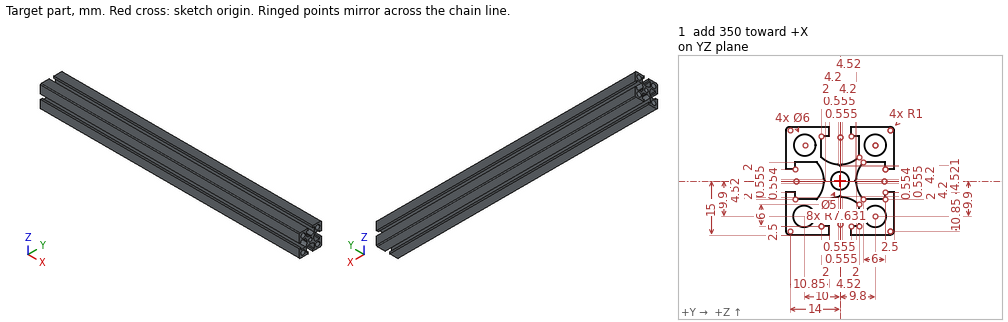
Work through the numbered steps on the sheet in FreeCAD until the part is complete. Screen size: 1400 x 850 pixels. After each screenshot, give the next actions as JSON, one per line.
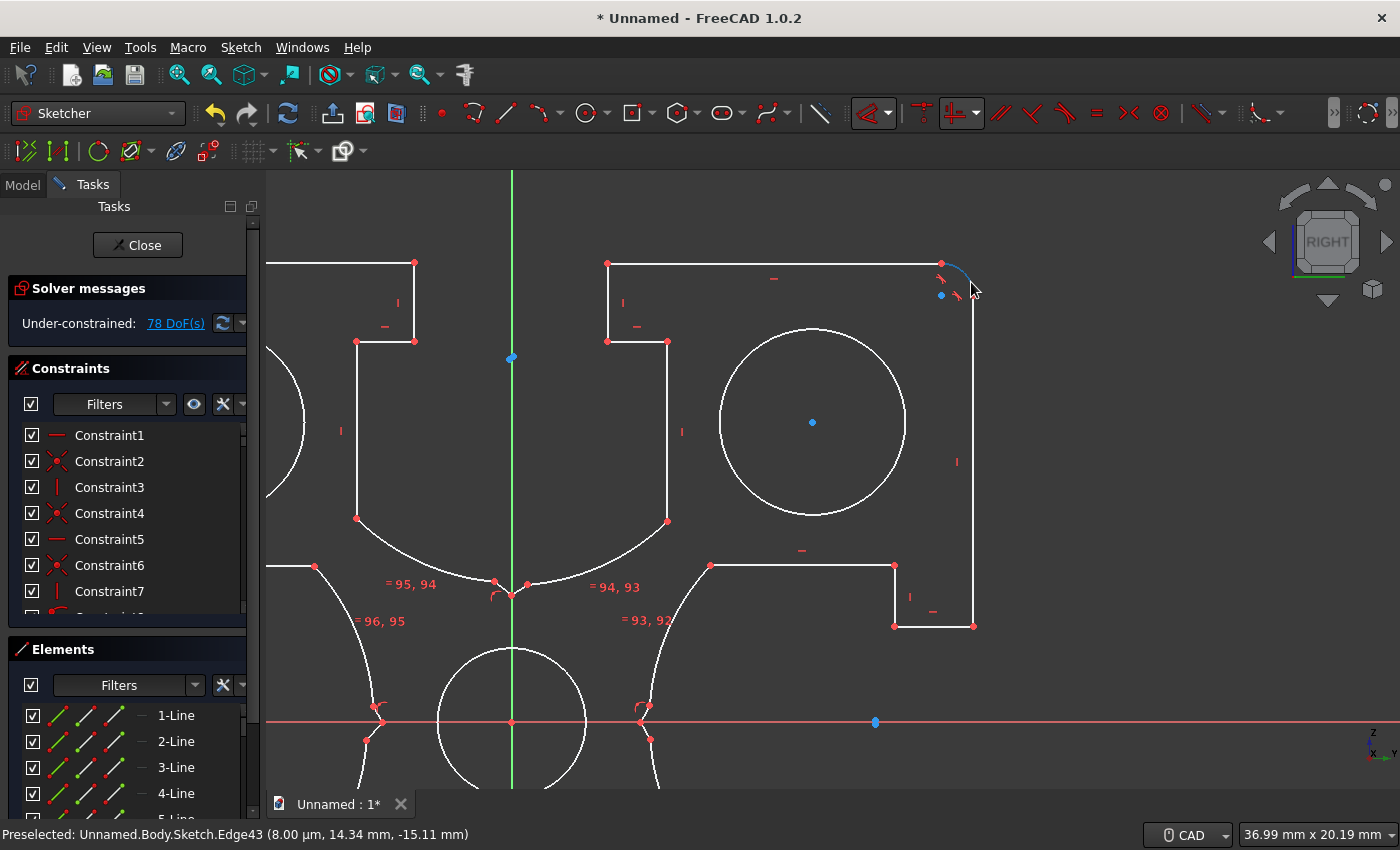
{"action": "left_click", "coordinate": [970, 281]}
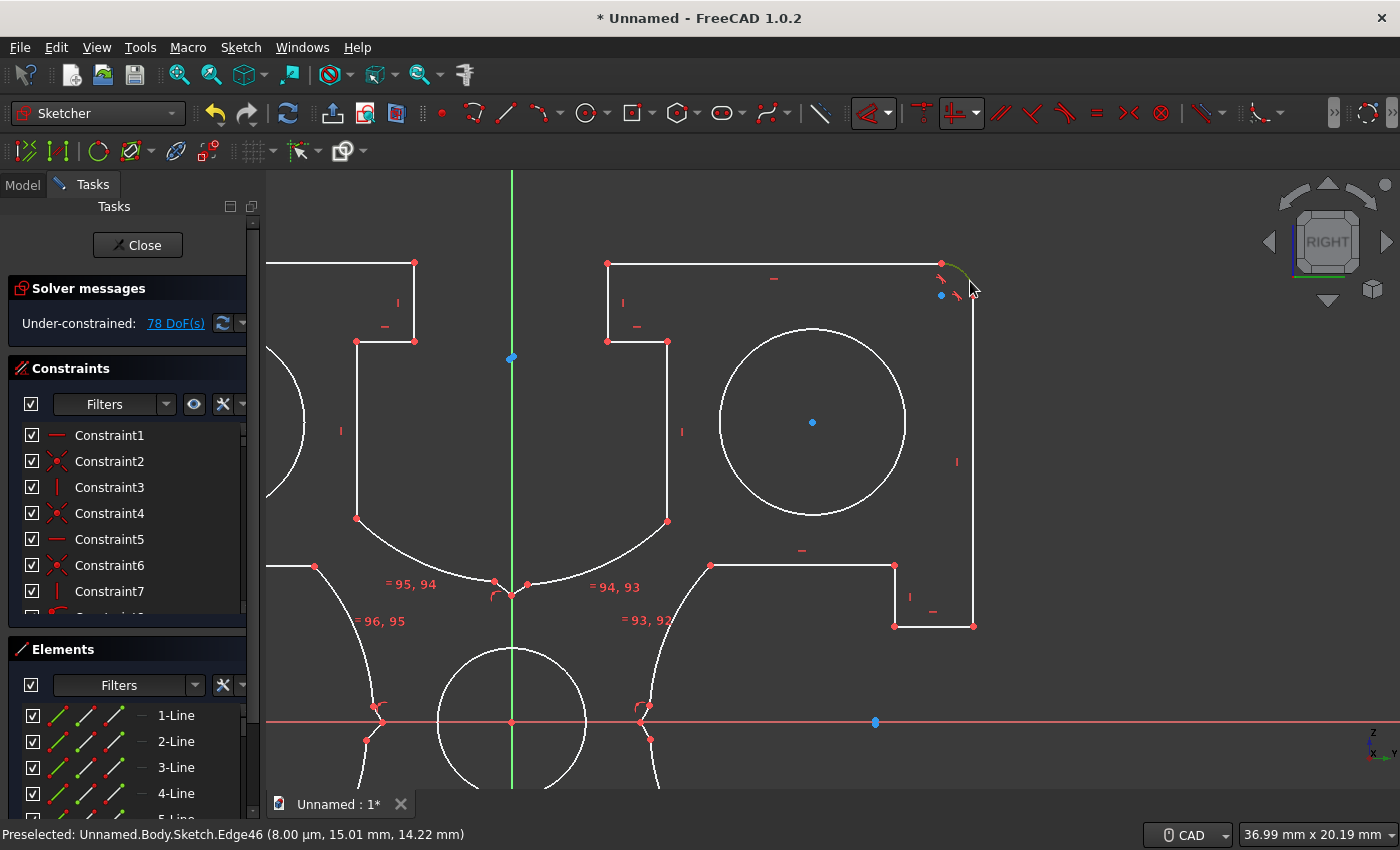
{"action": "scroll", "coordinate": [971, 281], "scroll_direction": "down", "scroll_amount": 4}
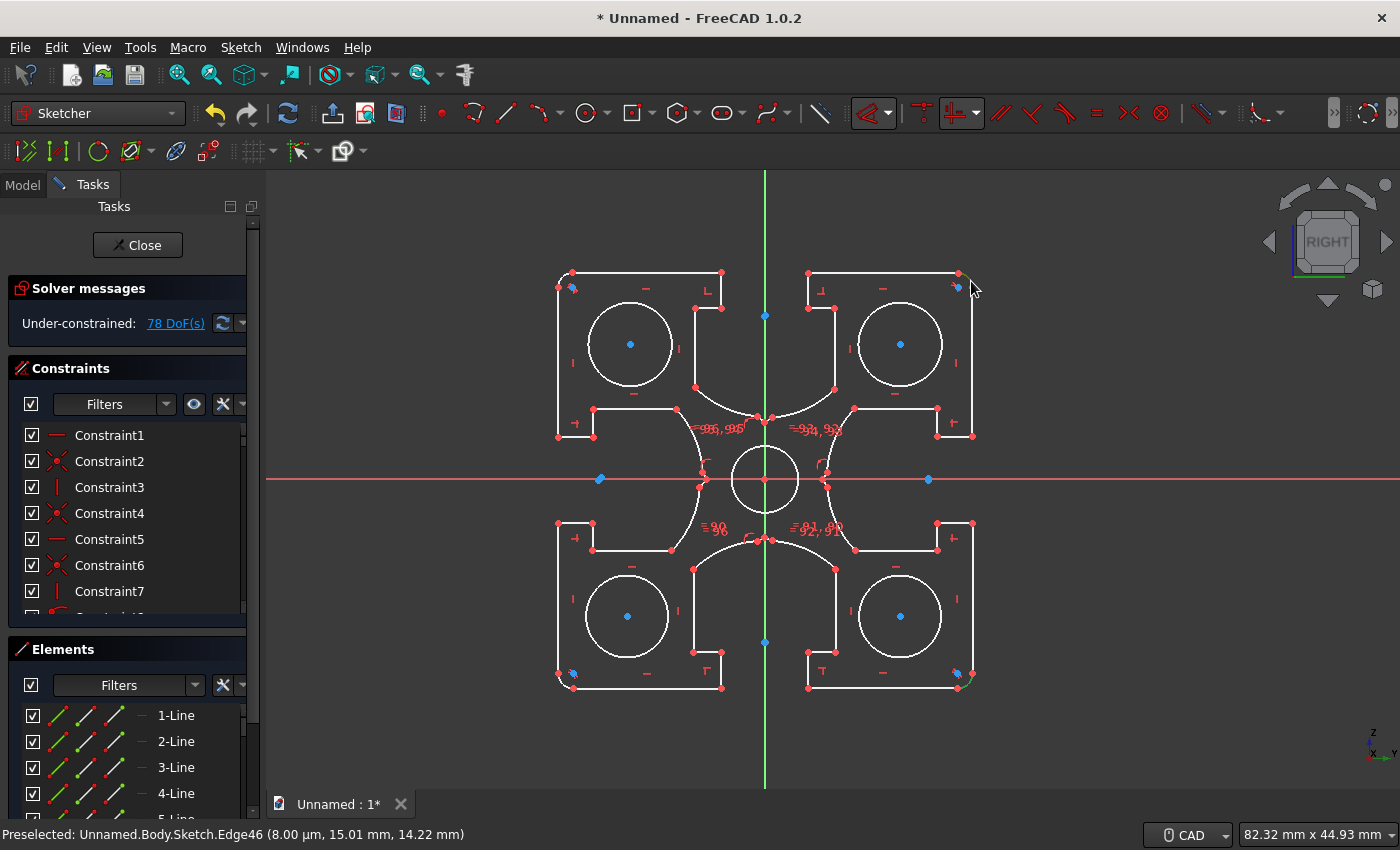
{"action": "scroll", "coordinate": [566, 274], "scroll_direction": "up", "scroll_amount": 4}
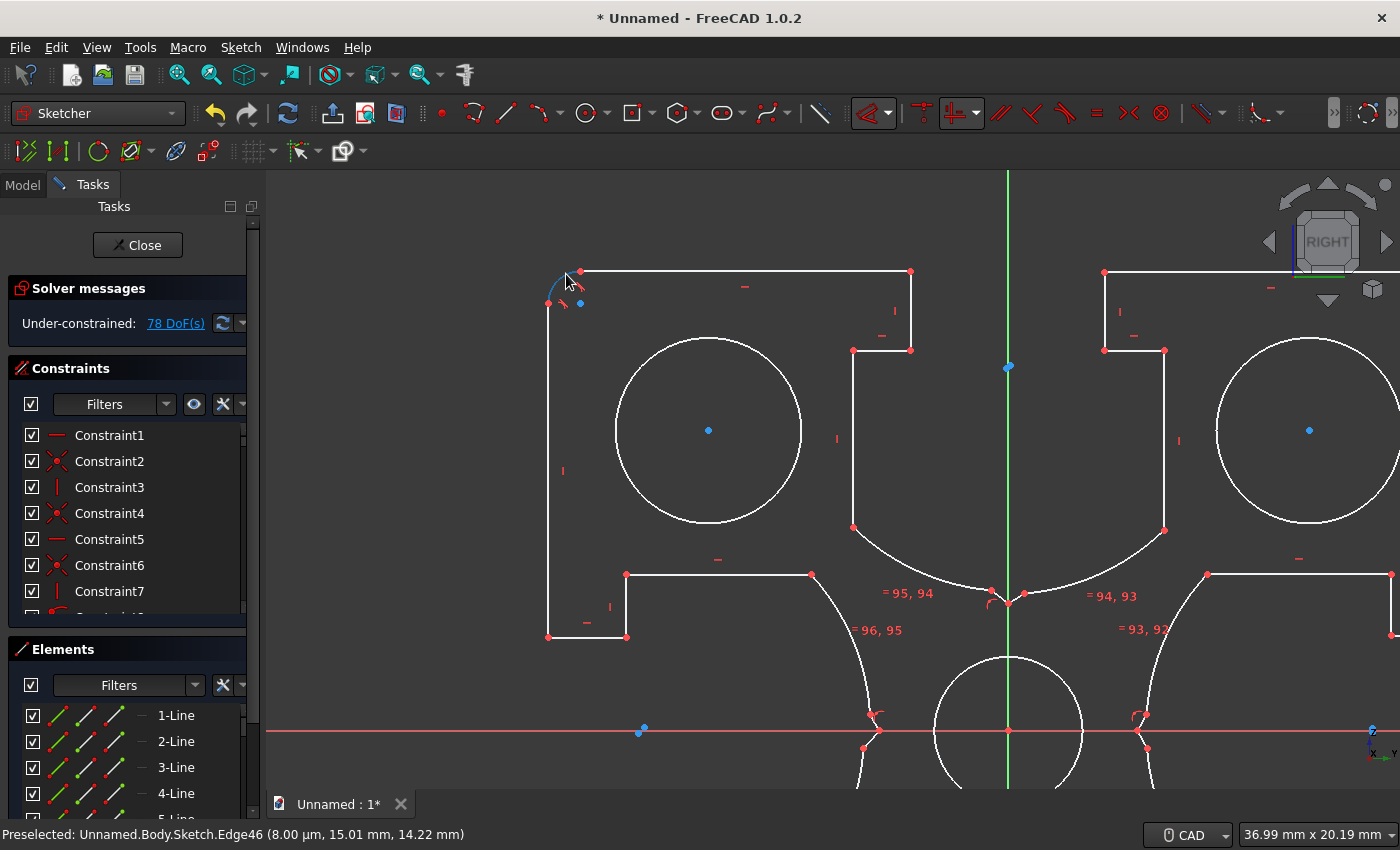
{"action": "left_click", "coordinate": [566, 275]}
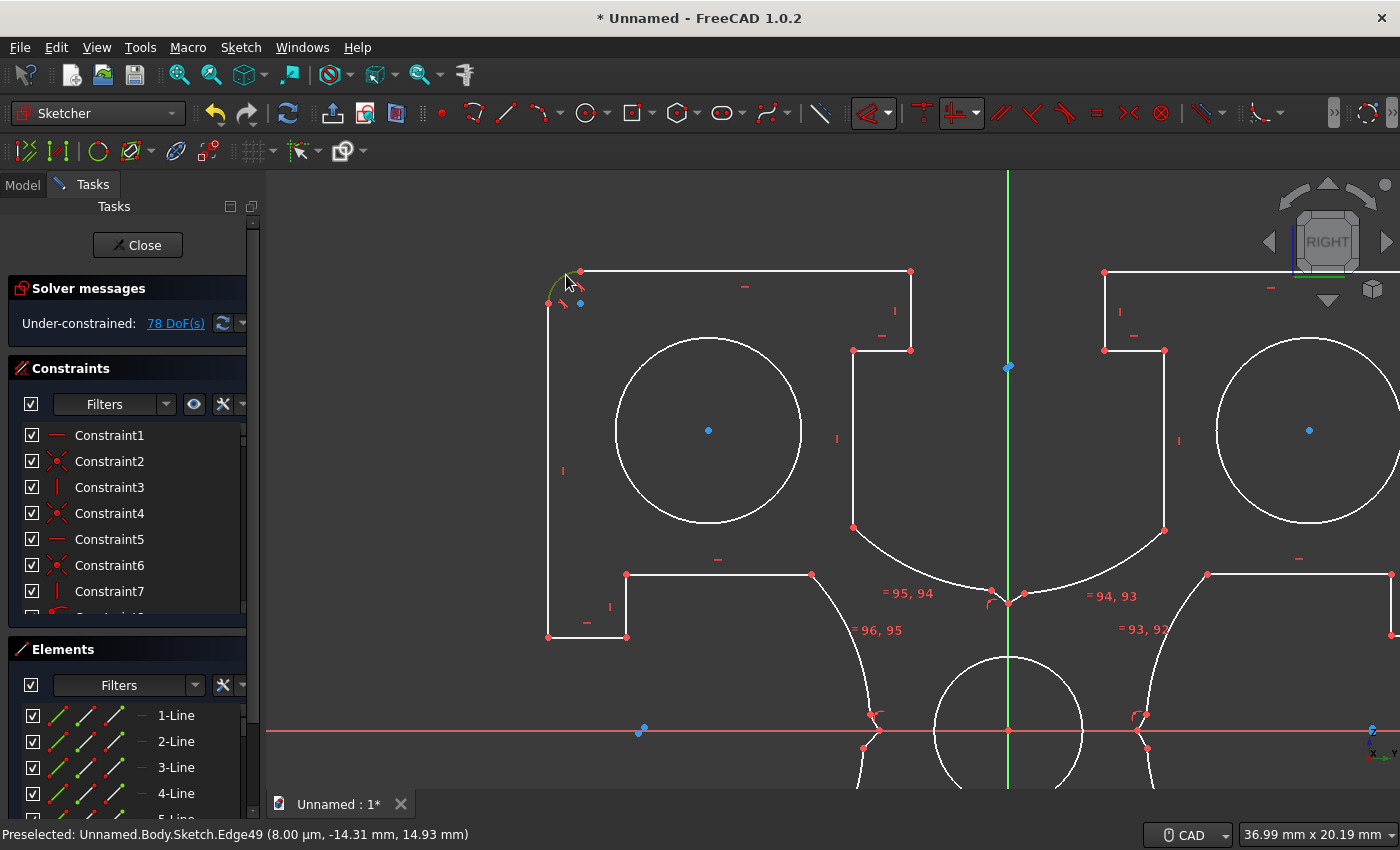
{"action": "scroll", "coordinate": [565, 274], "scroll_direction": "down", "scroll_amount": 4}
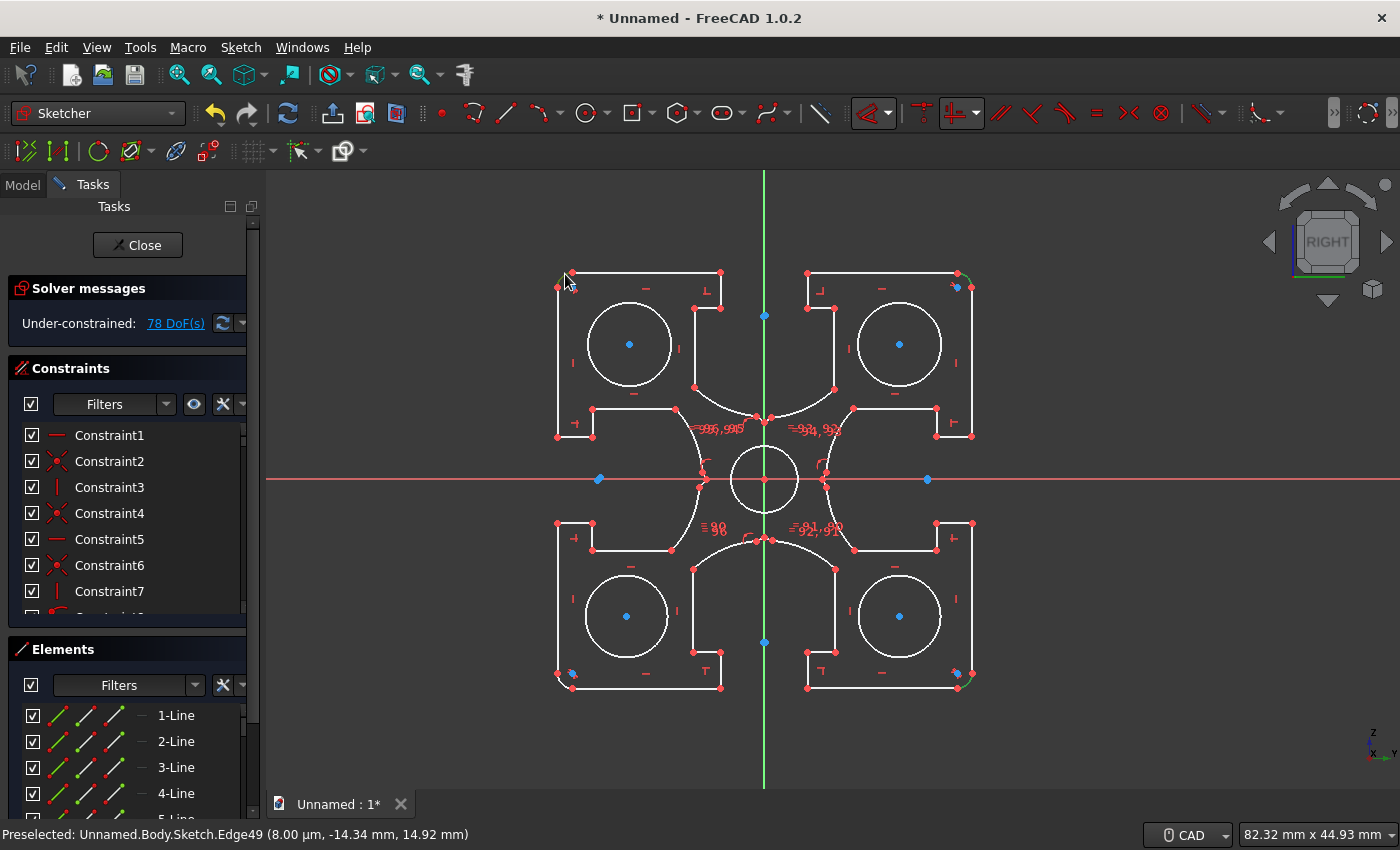
{"action": "scroll", "coordinate": [559, 680], "scroll_direction": "up", "scroll_amount": 4}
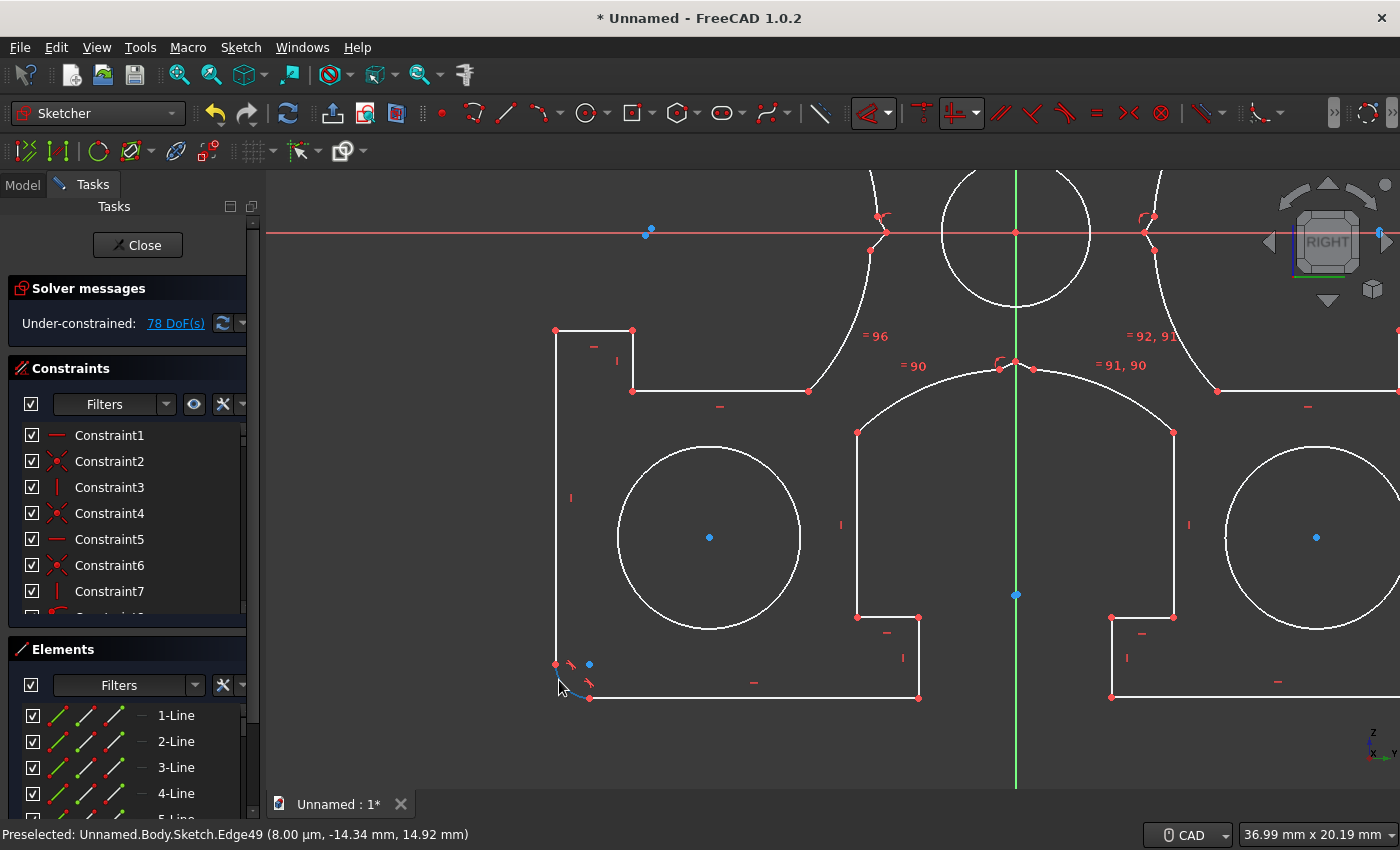
{"action": "left_click", "coordinate": [559, 680]}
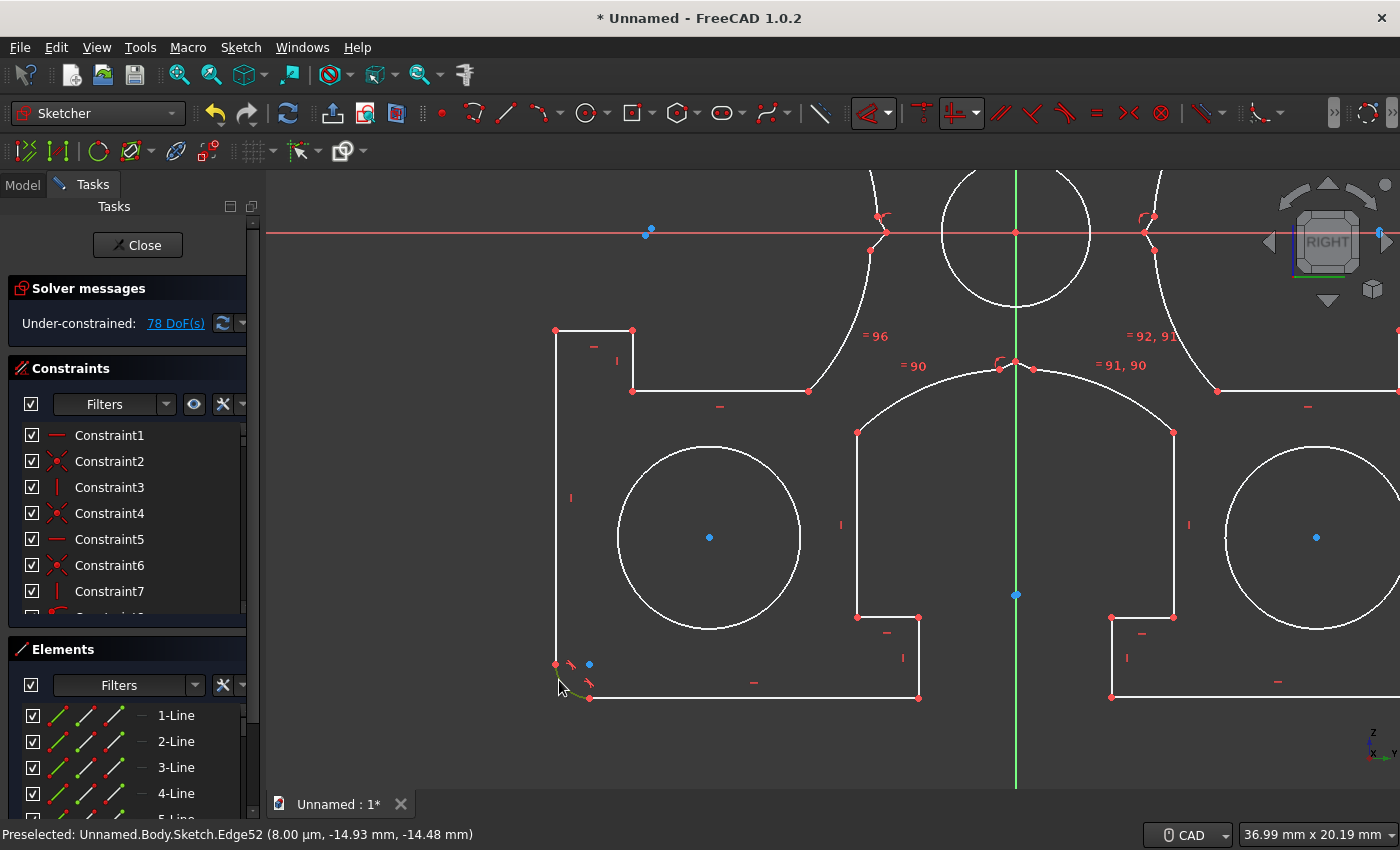
{"action": "left_click", "coordinate": [1098, 114]}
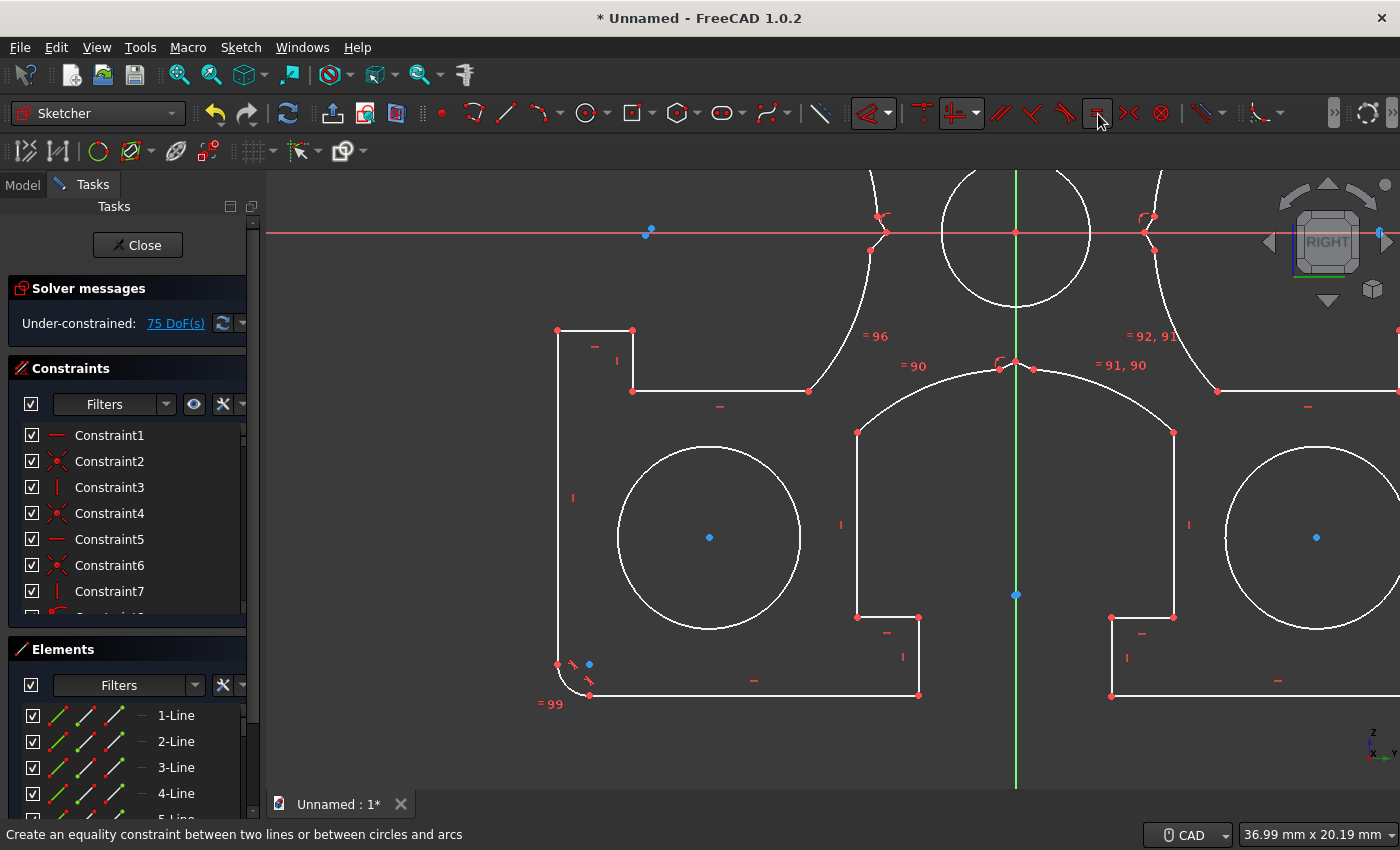
{"action": "left_click", "coordinate": [773, 473]}